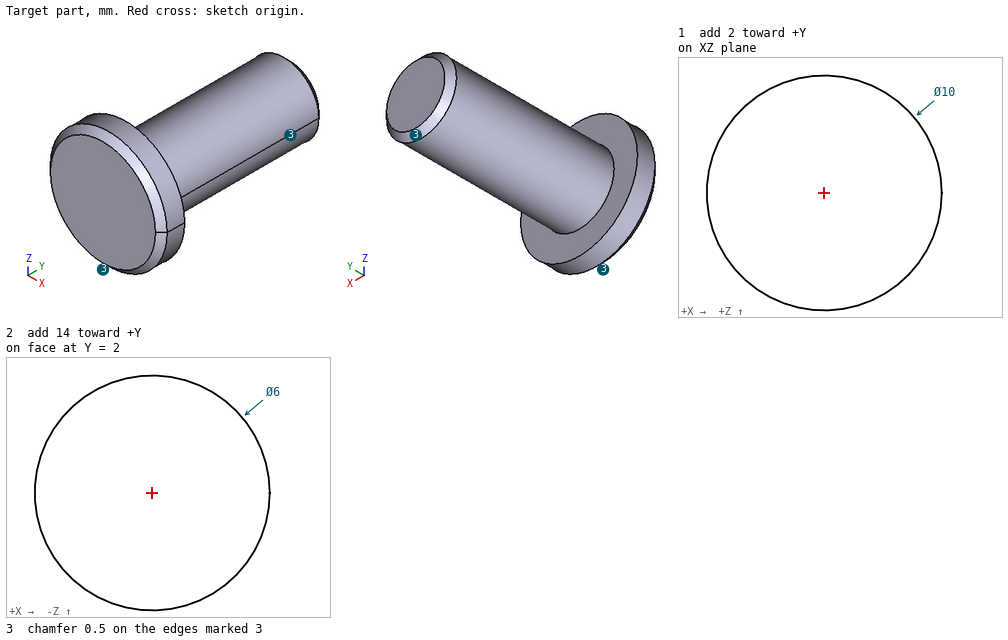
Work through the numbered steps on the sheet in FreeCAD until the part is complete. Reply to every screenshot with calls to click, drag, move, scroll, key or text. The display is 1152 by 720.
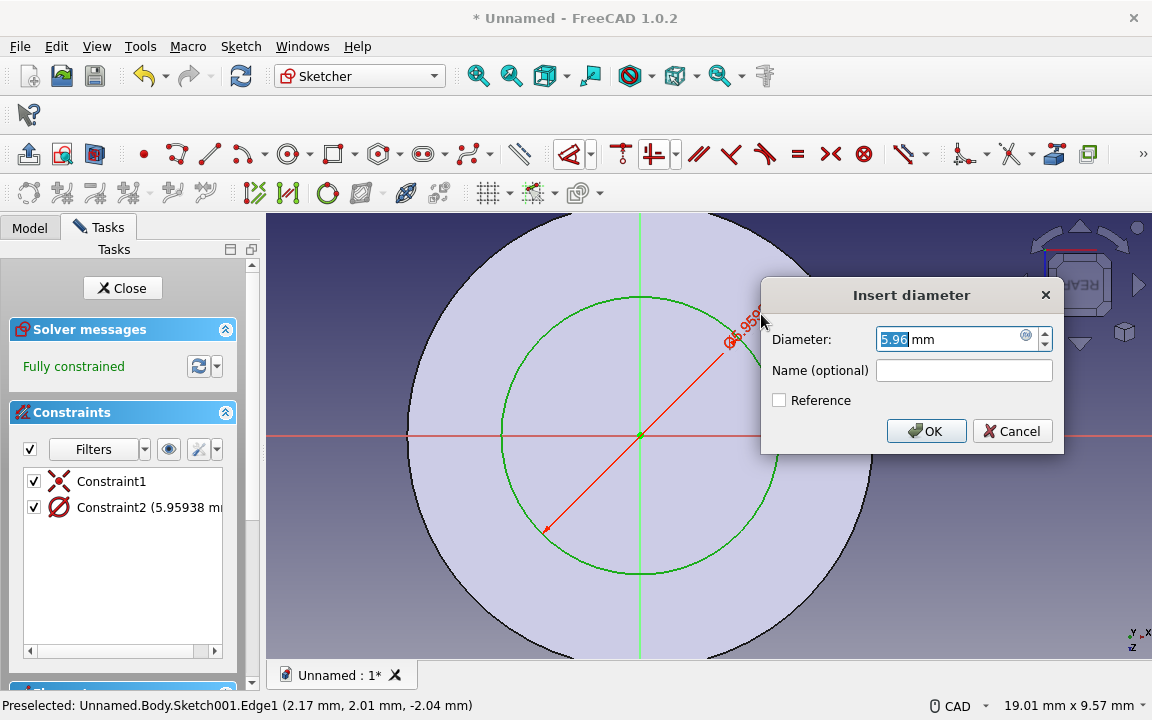
text(6)
key(Return)
key(Escape)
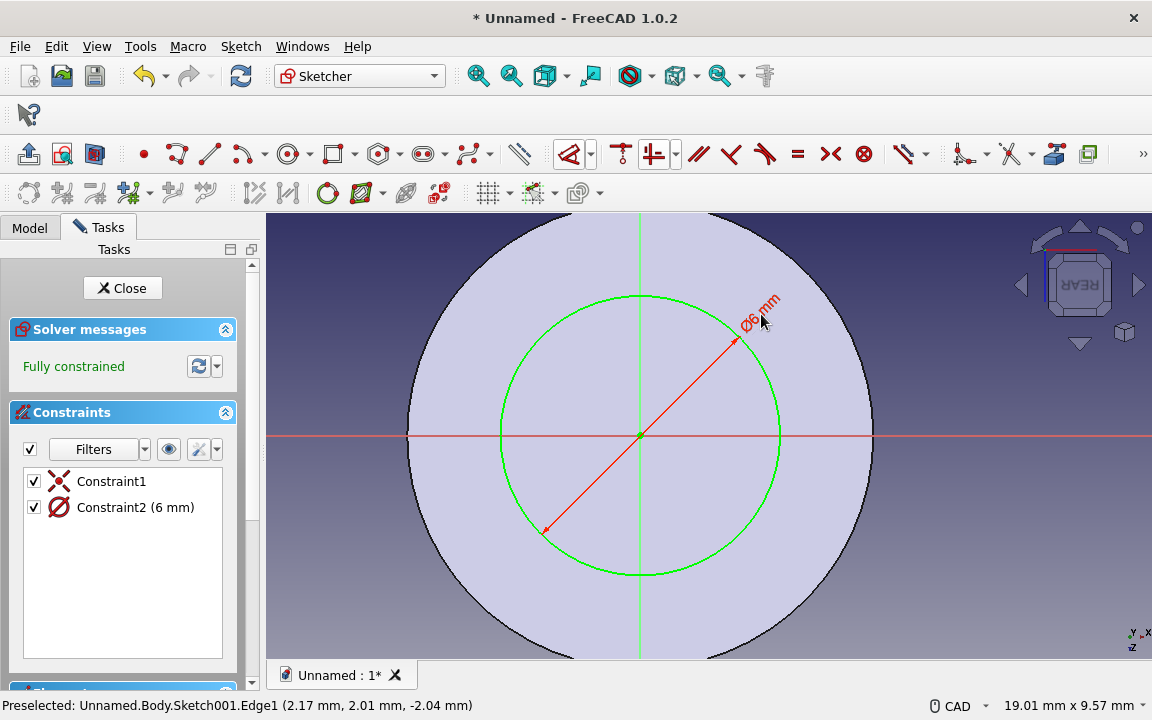
click(123, 288)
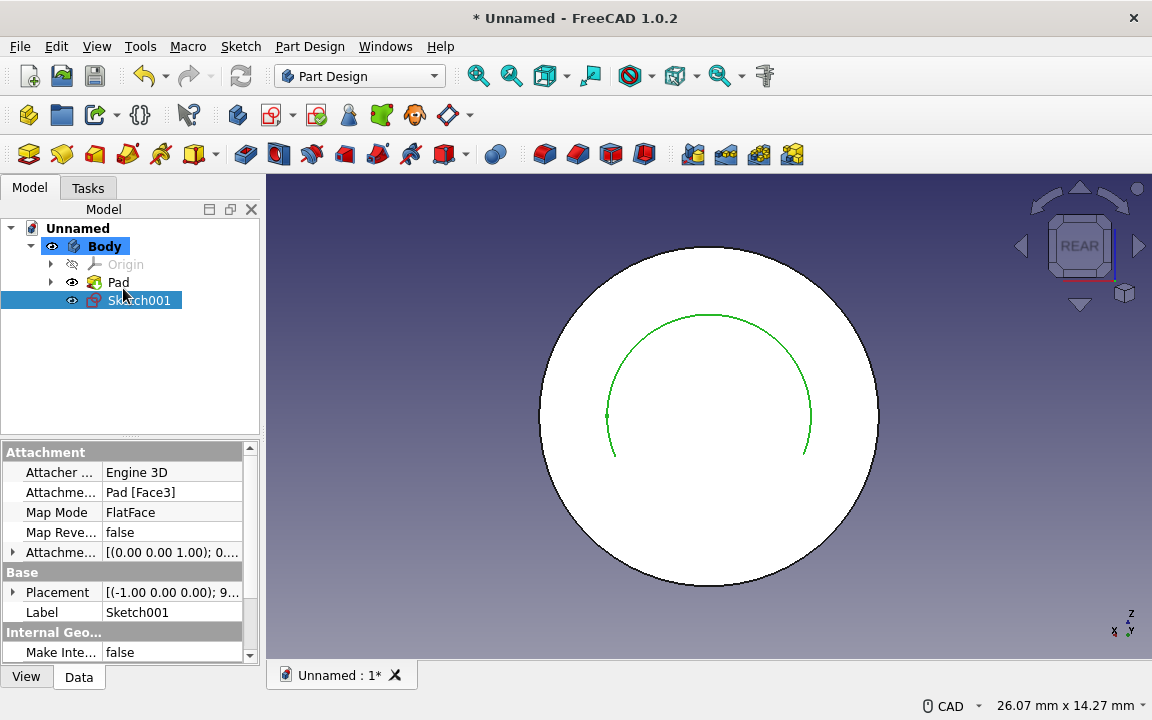
click(29, 154)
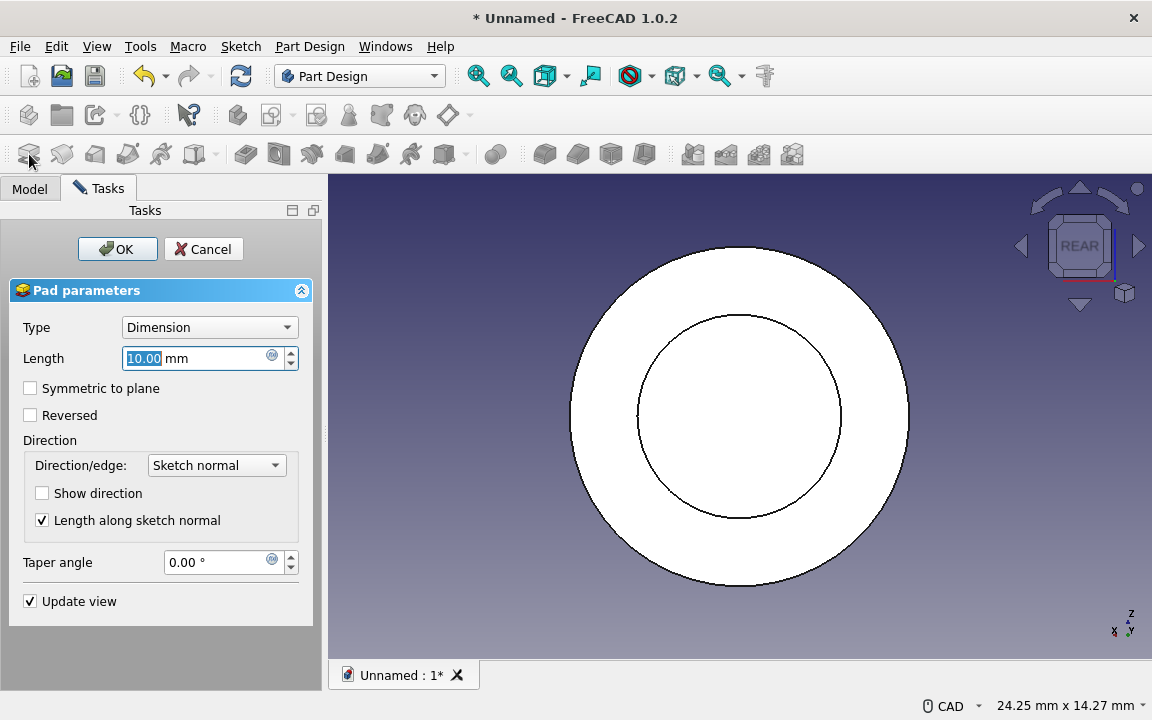
text(14)
key(Tab)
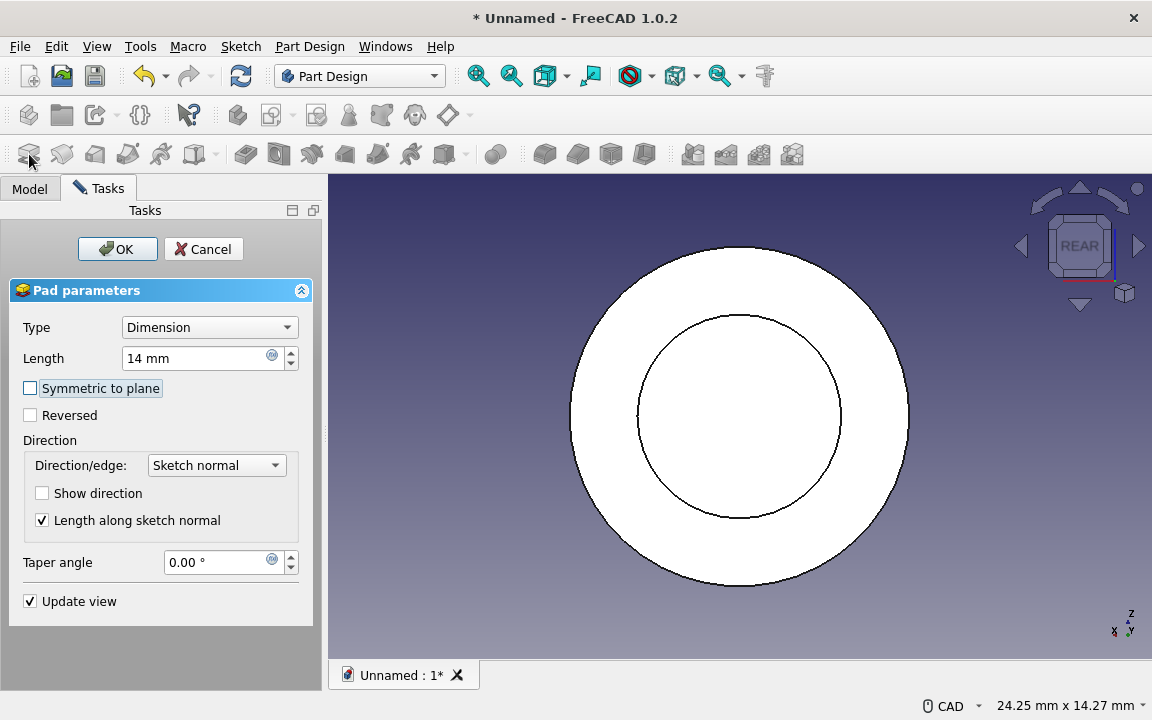
click(118, 249)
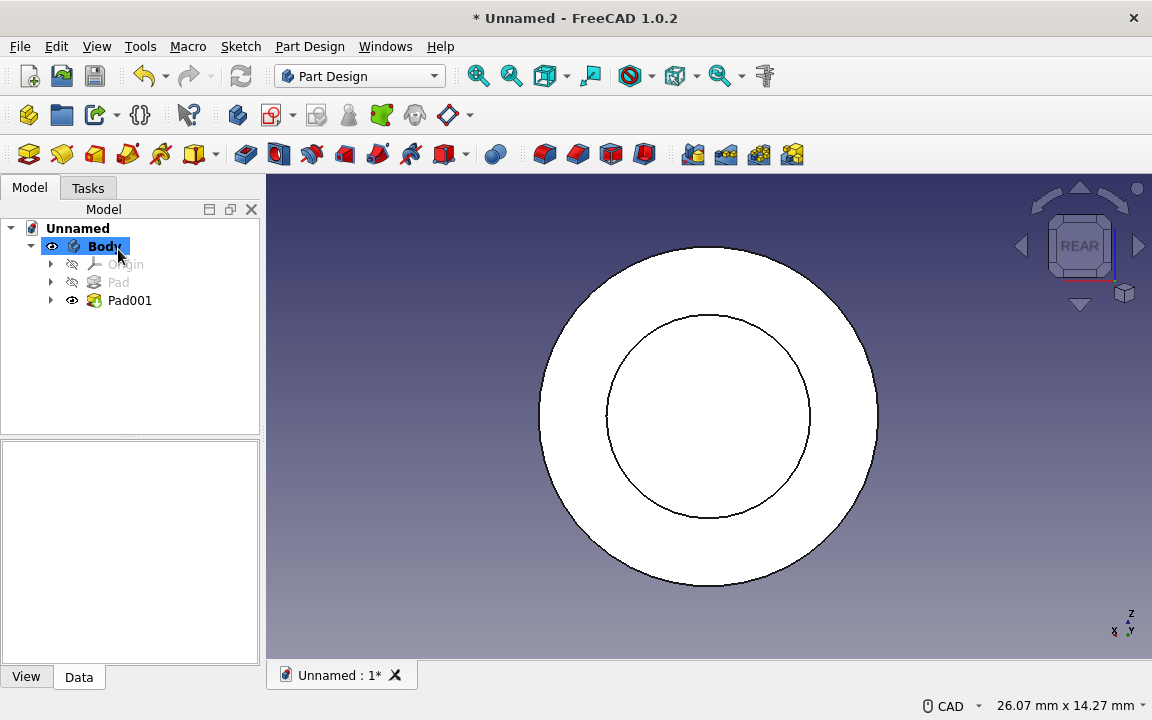
click(810, 416)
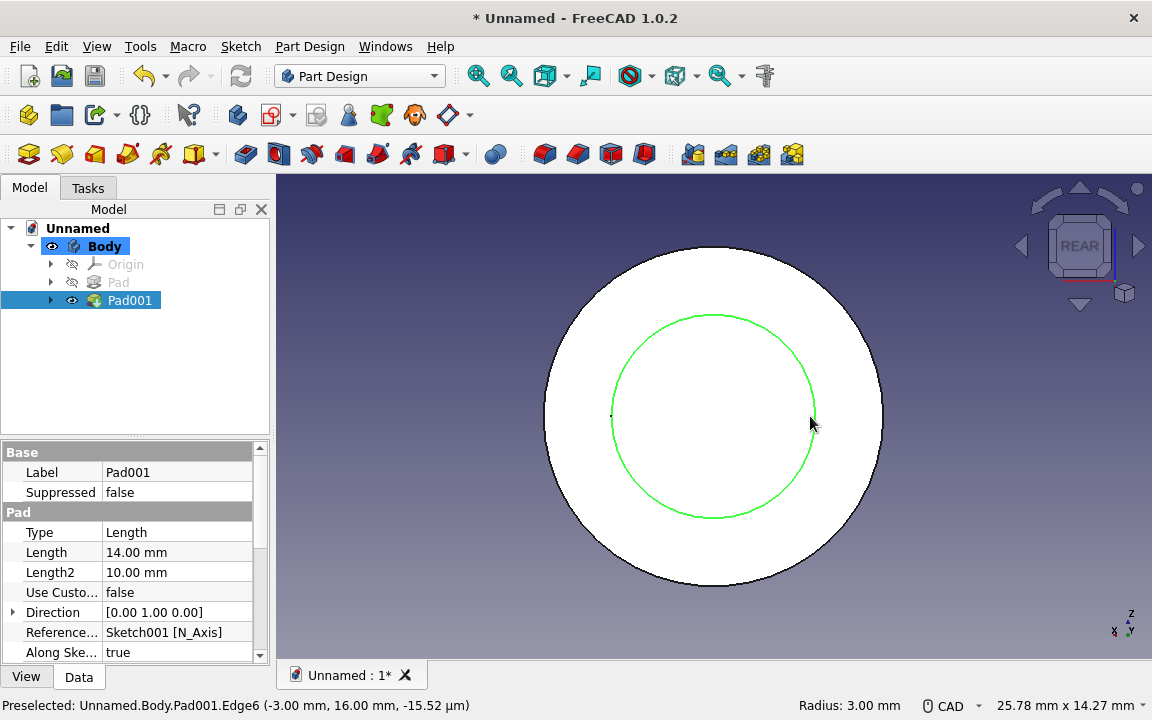
key(0)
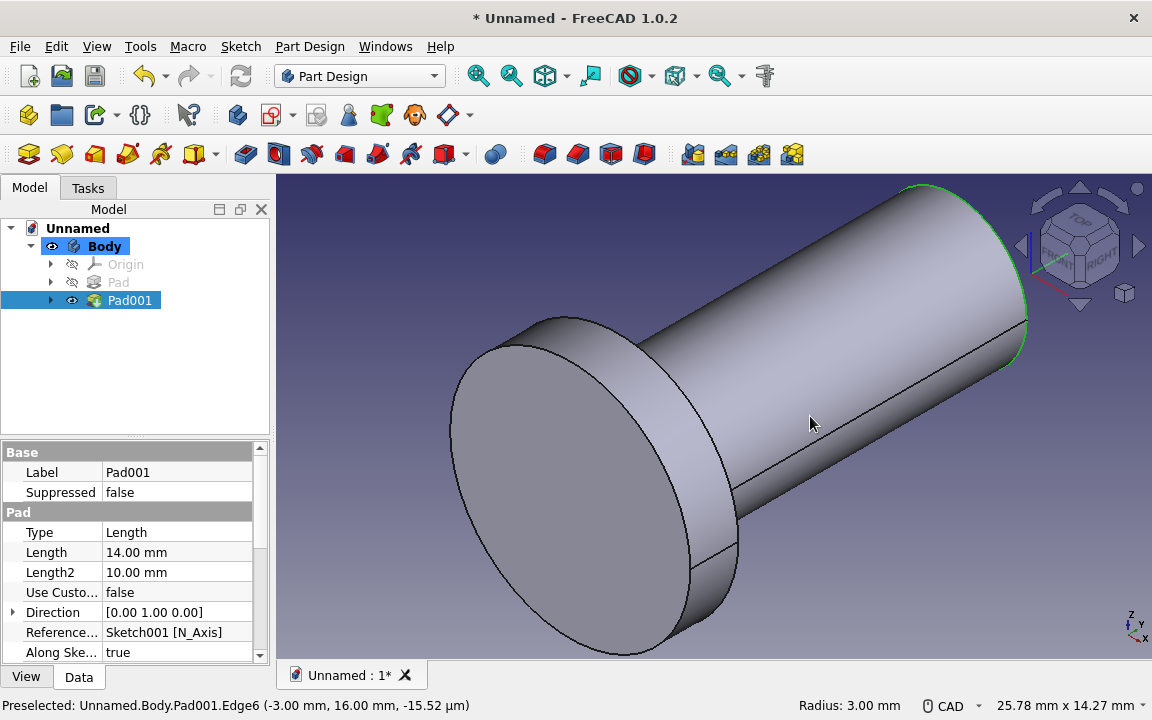
key(v)
key(f)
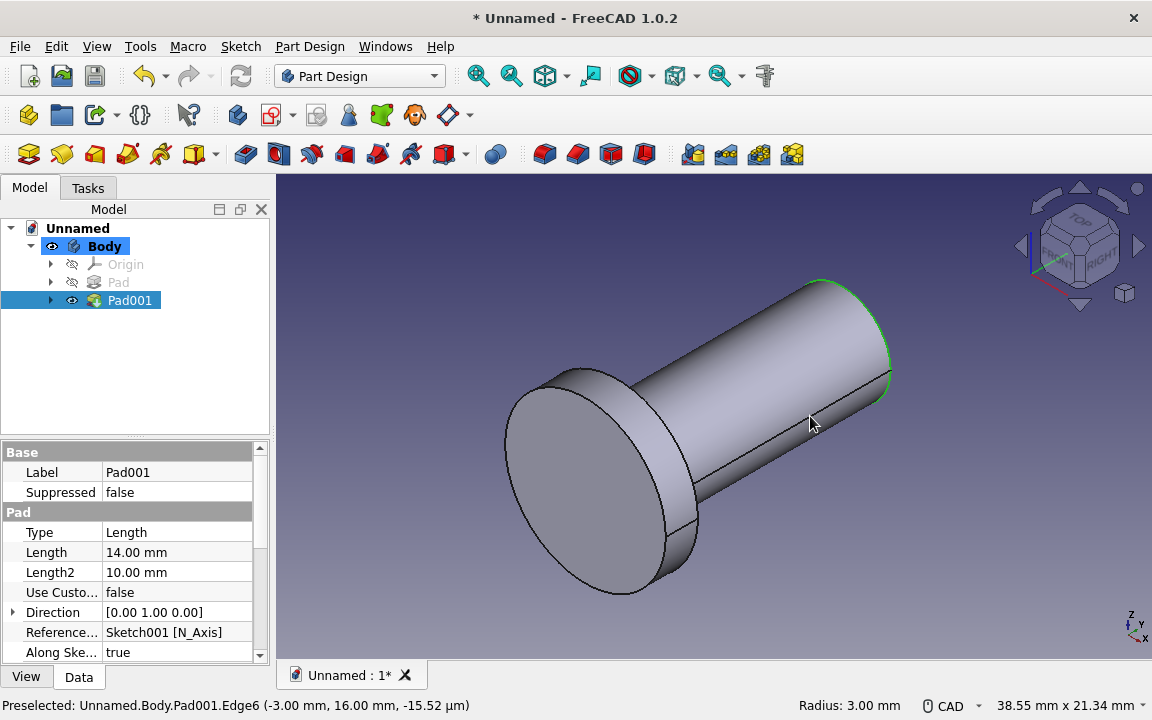
click(561, 387, ctrl)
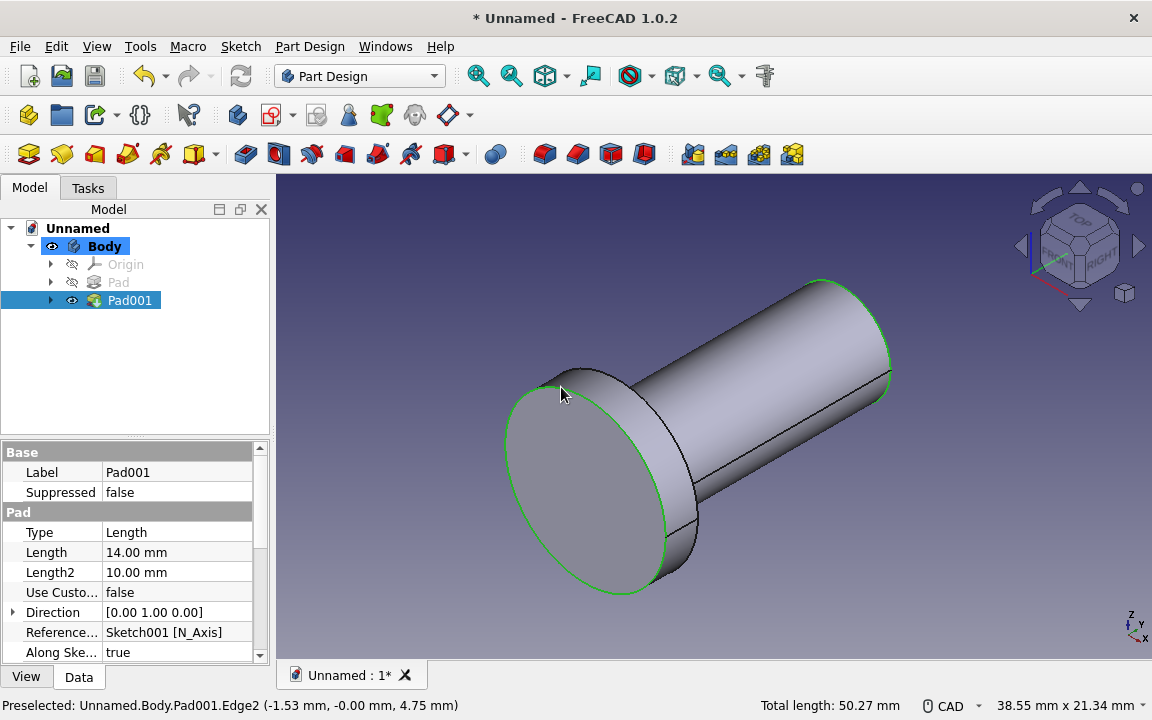
click(578, 154)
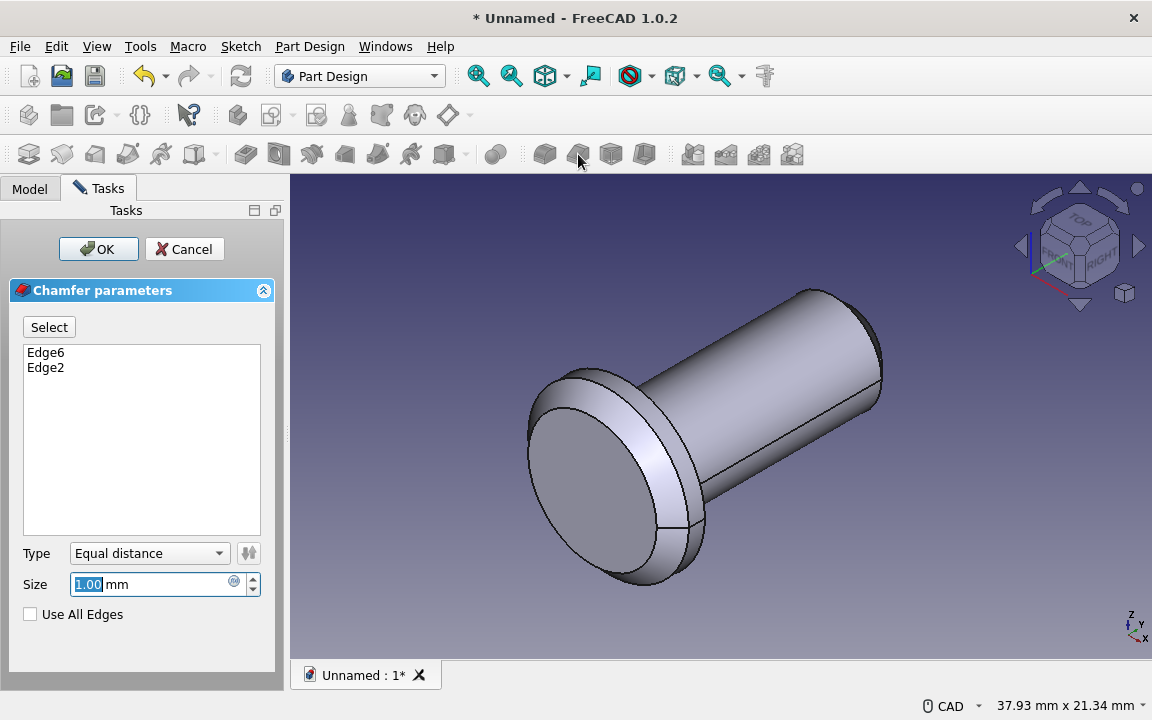
text(0.5)
key(Tab)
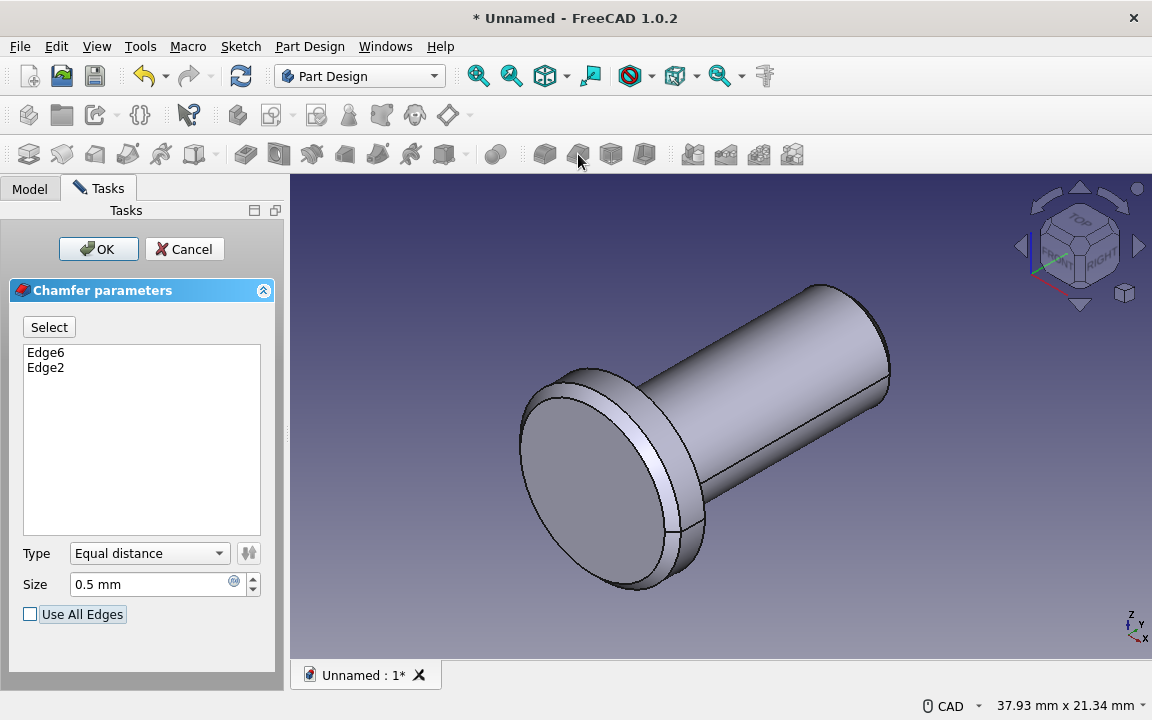
click(99, 249)